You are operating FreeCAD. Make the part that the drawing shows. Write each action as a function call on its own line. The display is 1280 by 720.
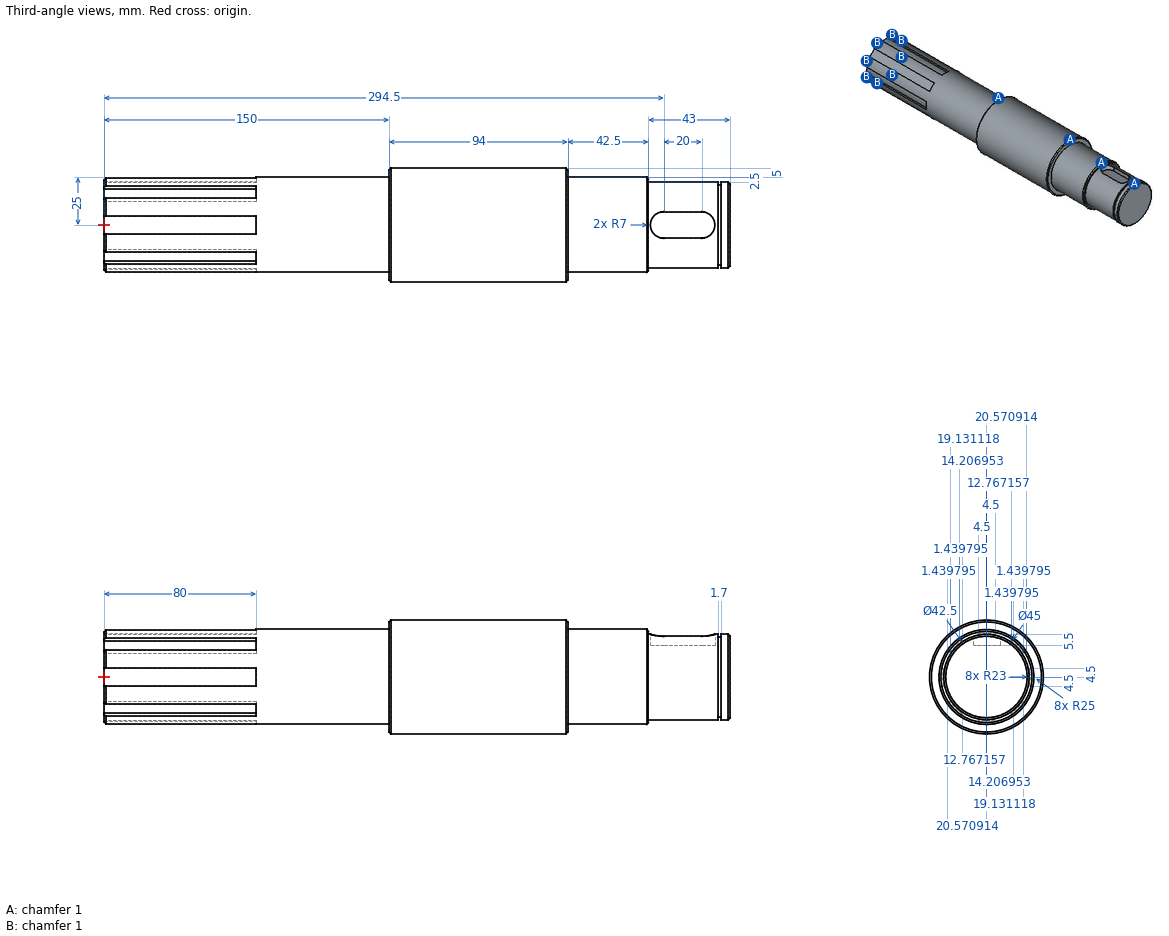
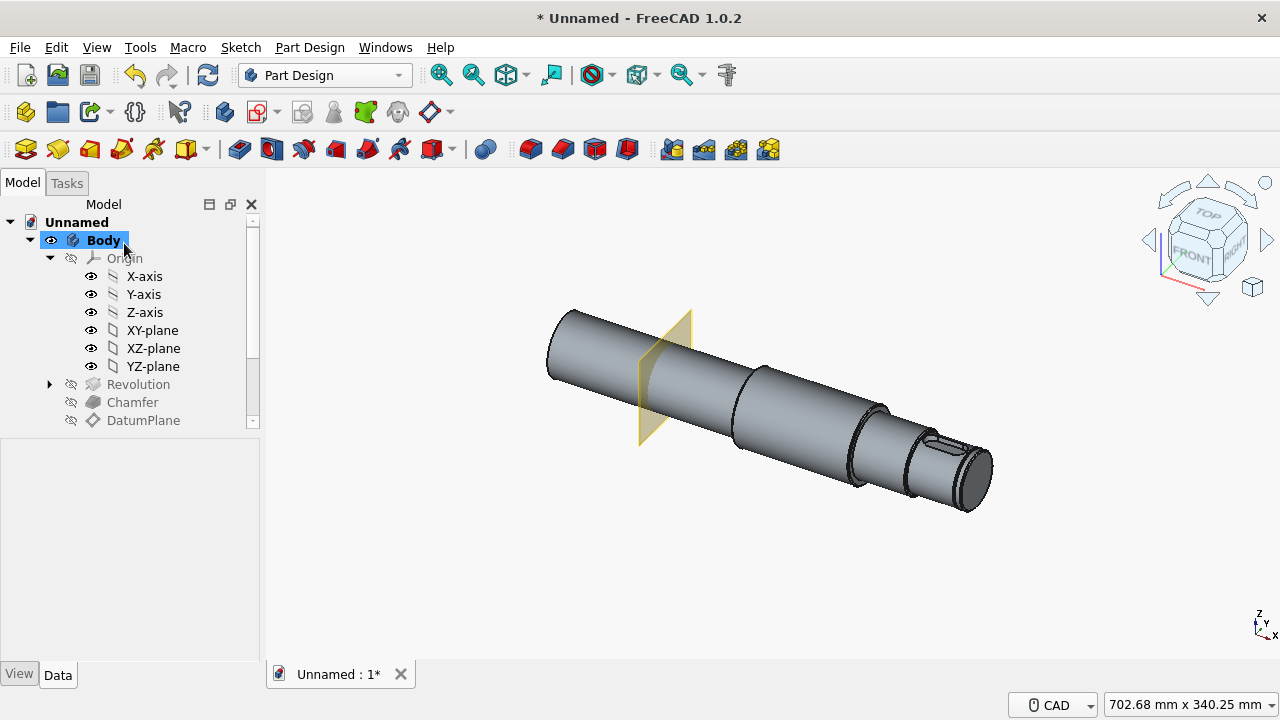
scroll(100, 326, down, 3)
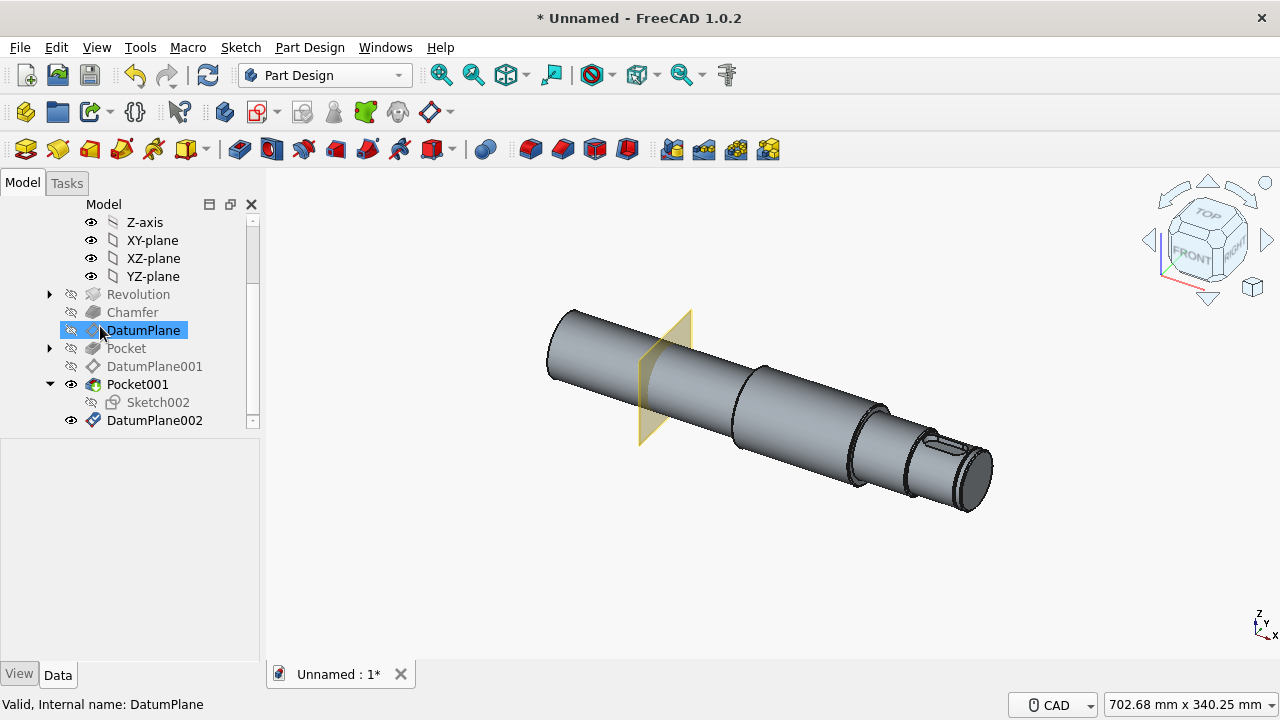
click(116, 420)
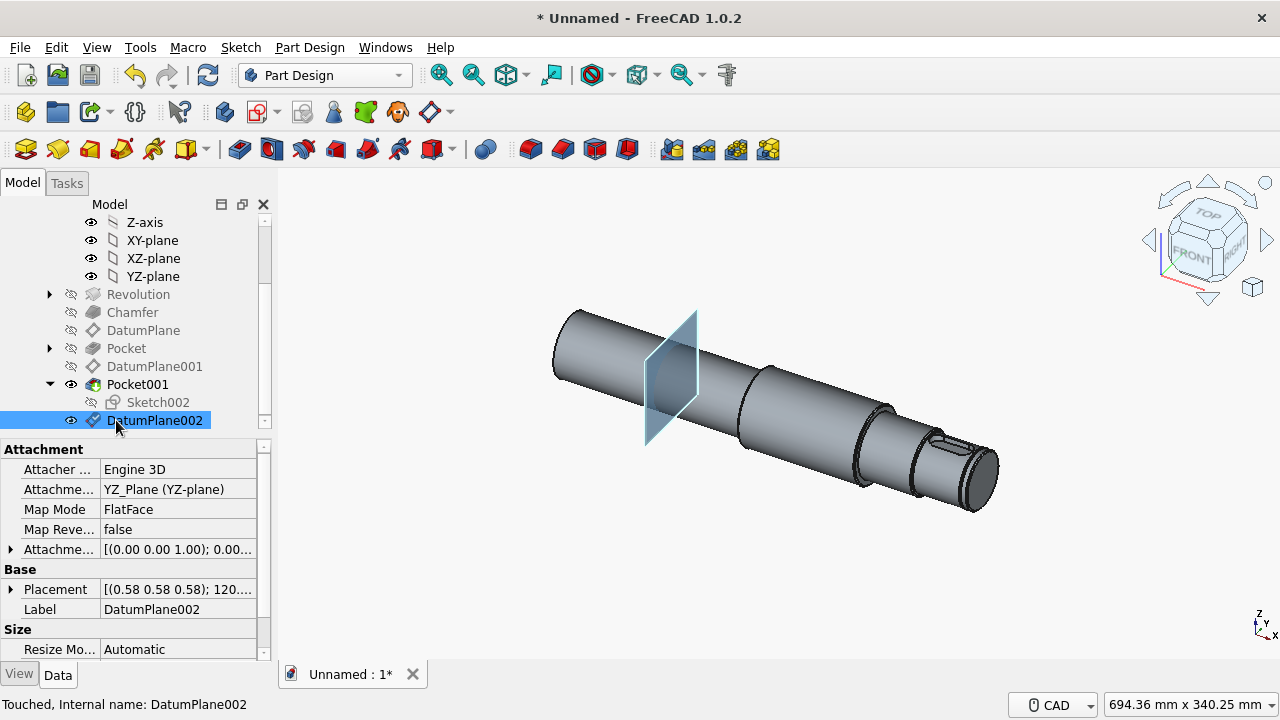
click(258, 112)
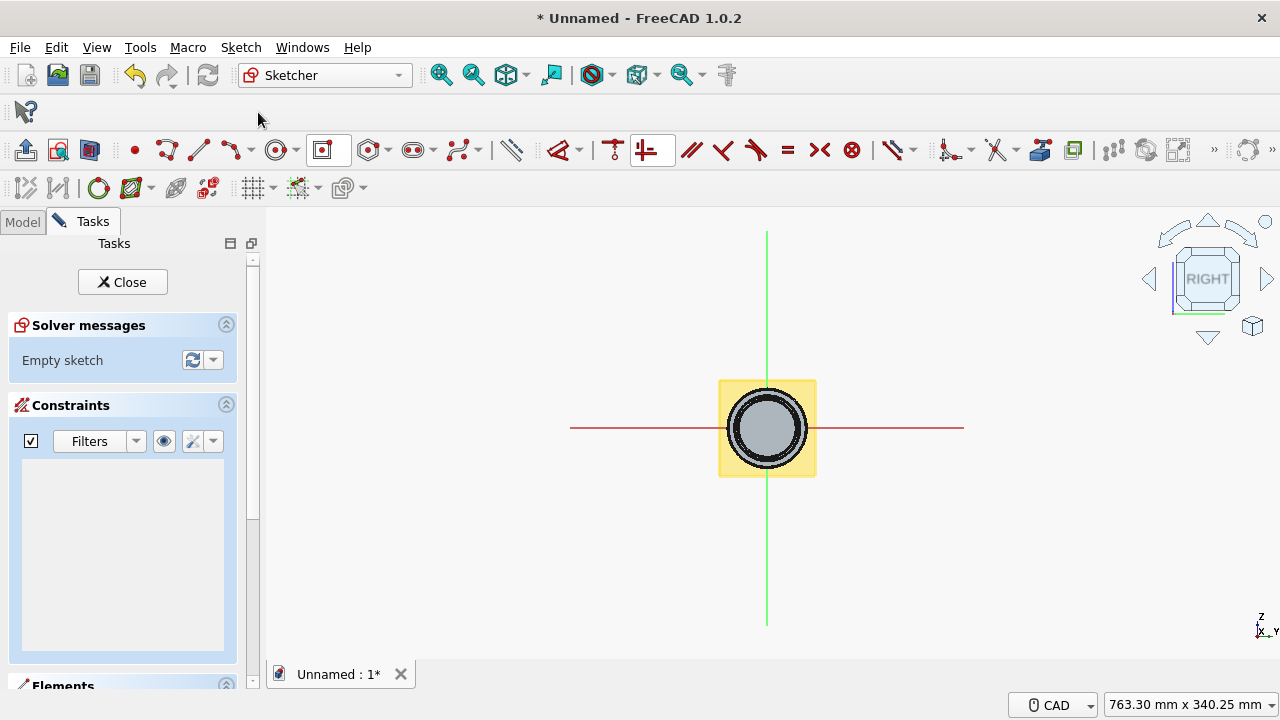
click(90, 150)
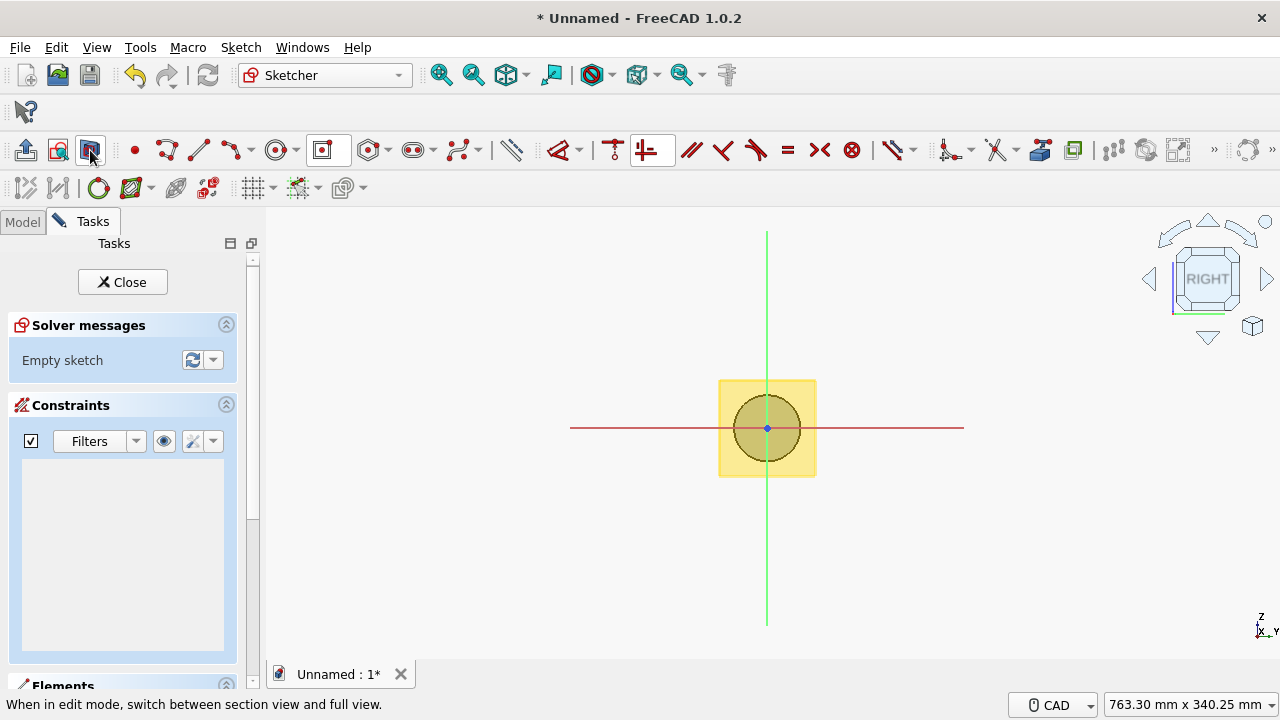
scroll(788, 427, up, 7)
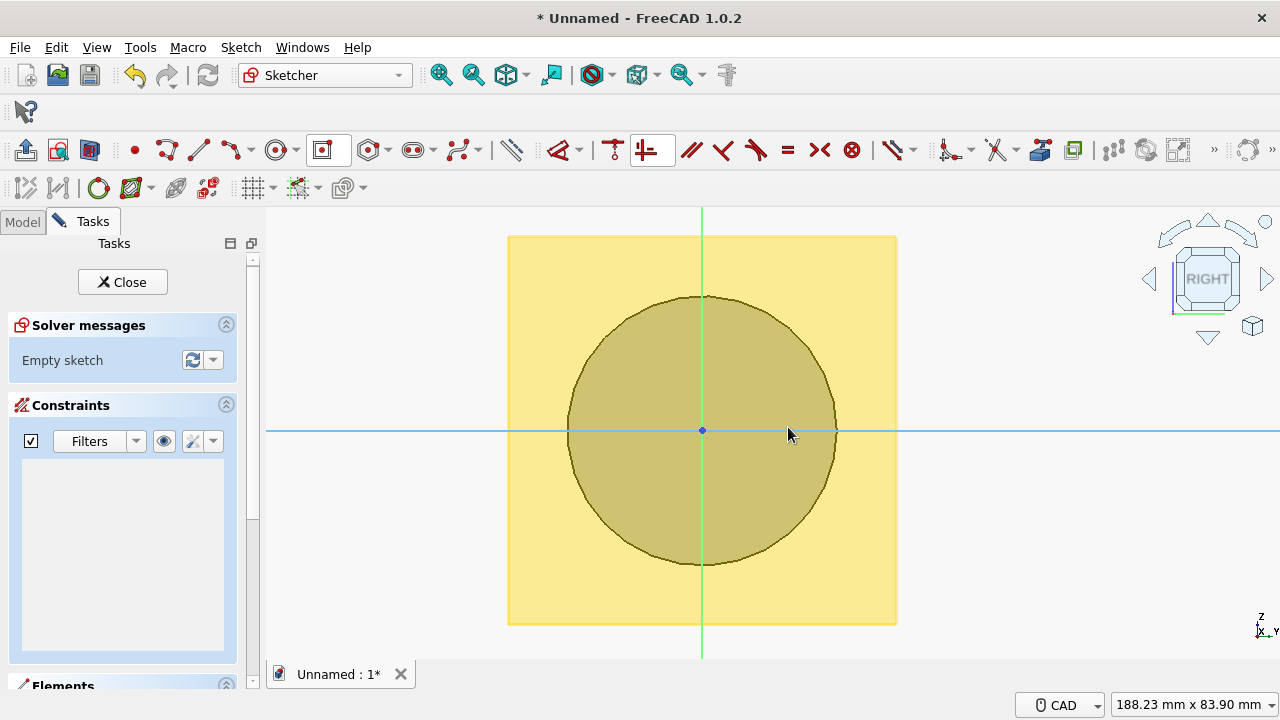
click(200, 150)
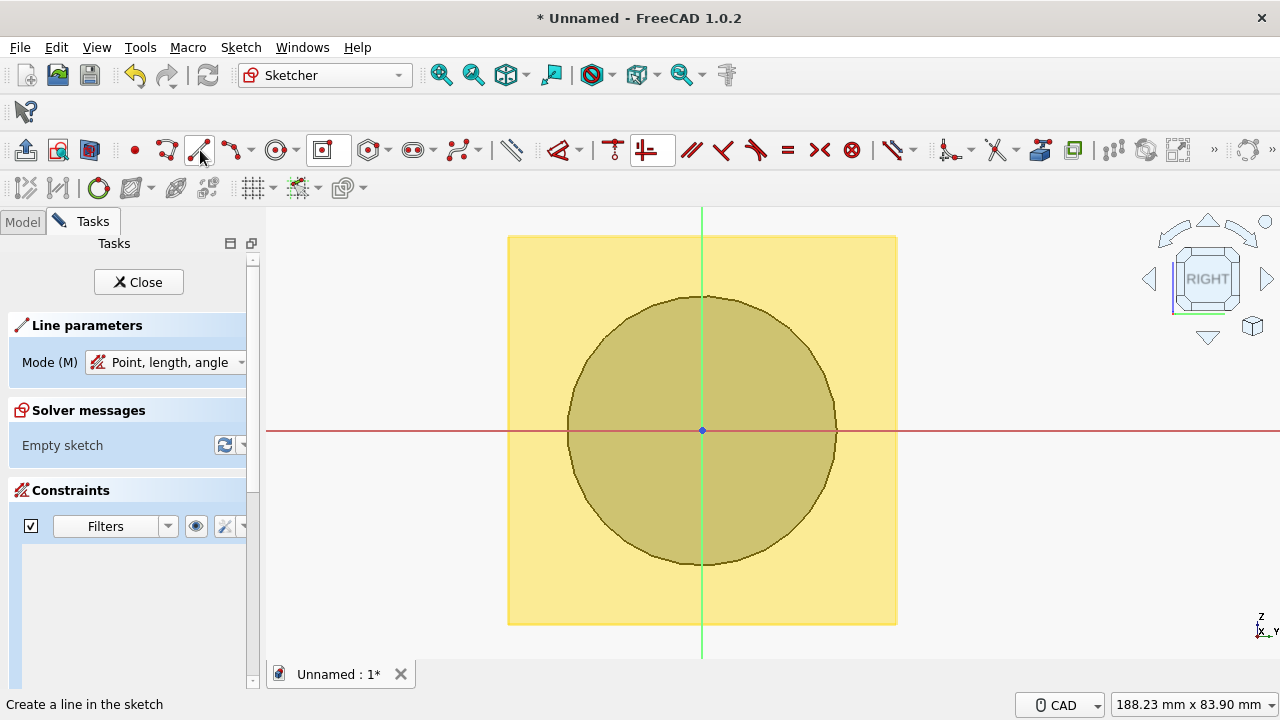
click(835, 455)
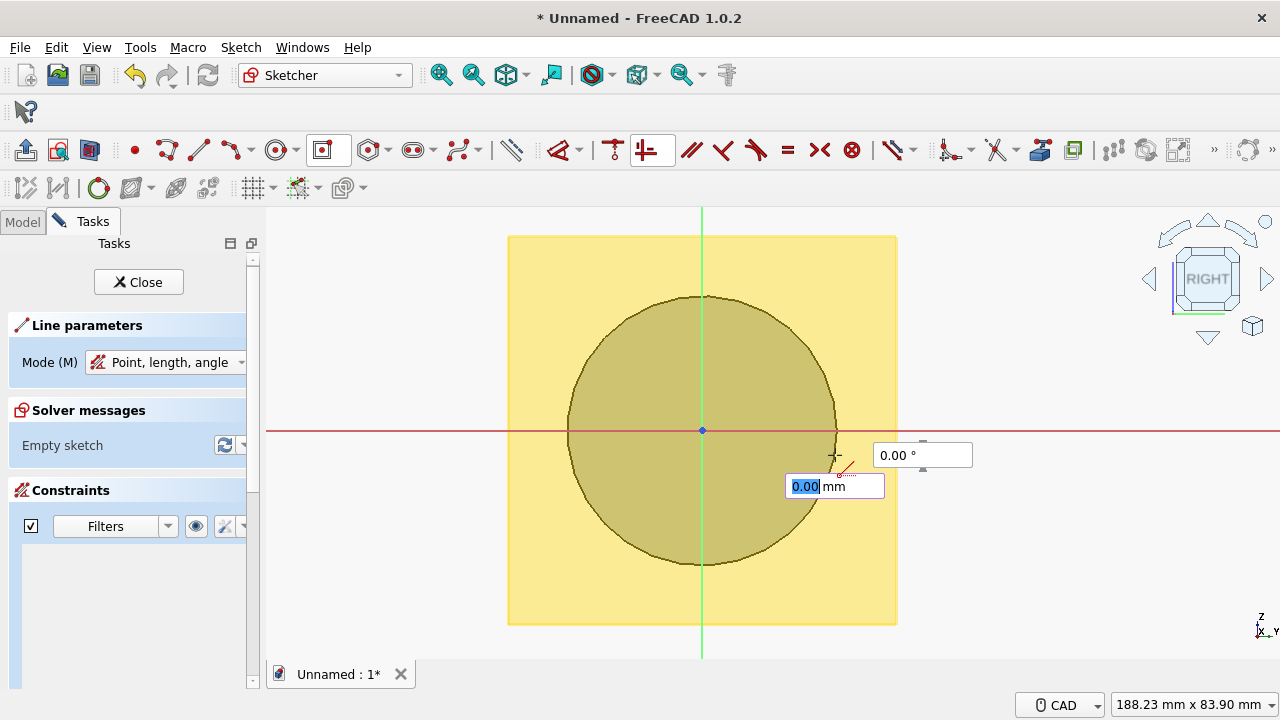
scroll(824, 455, up, 2)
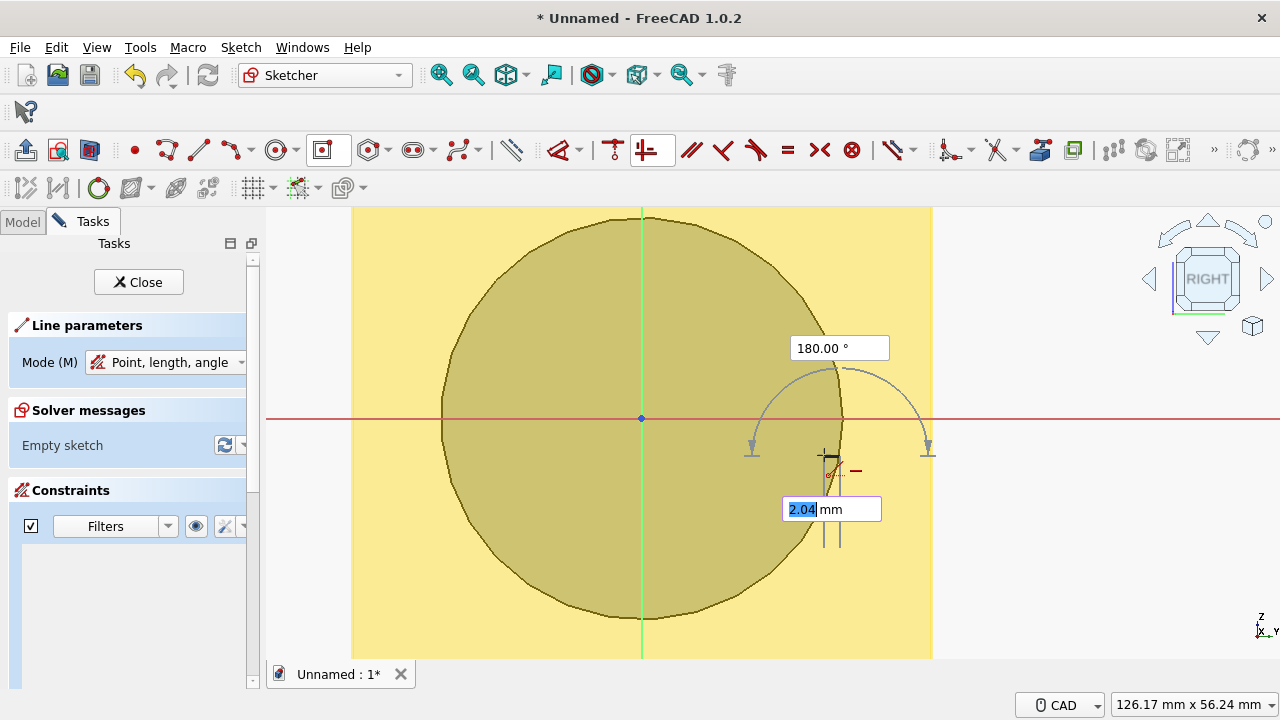
click(823, 455)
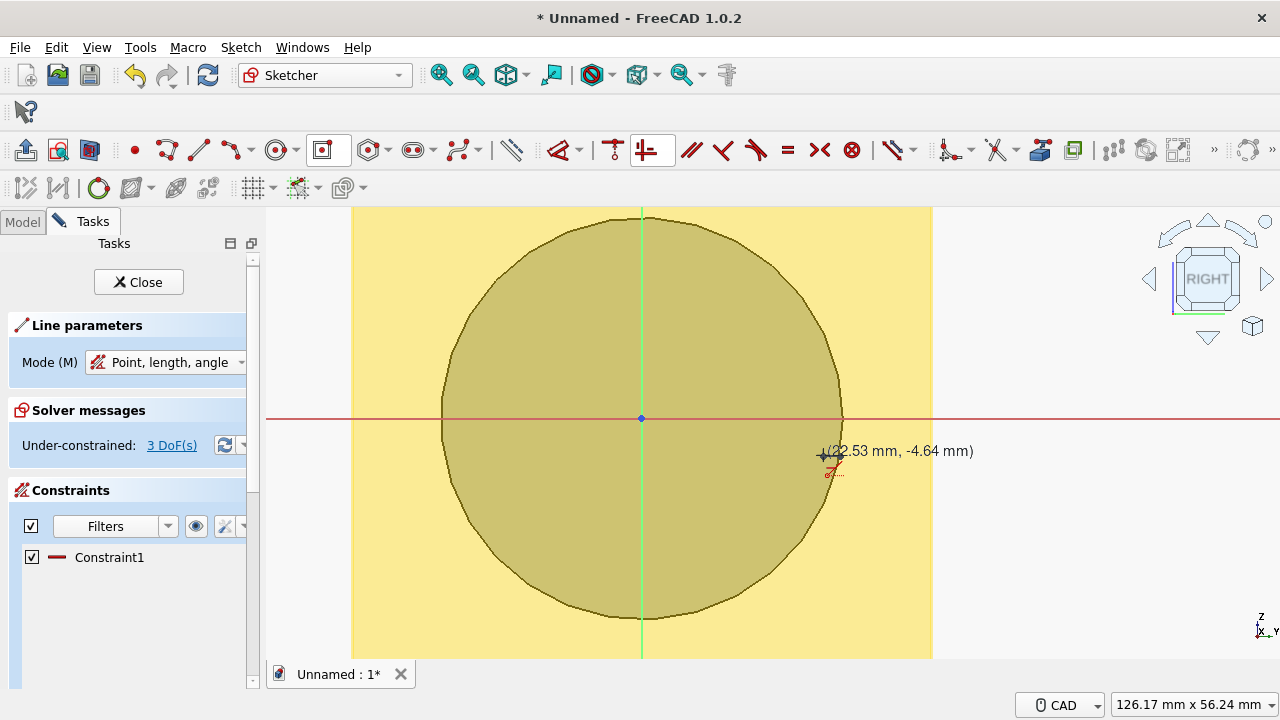
click(823, 383)
click(840, 383)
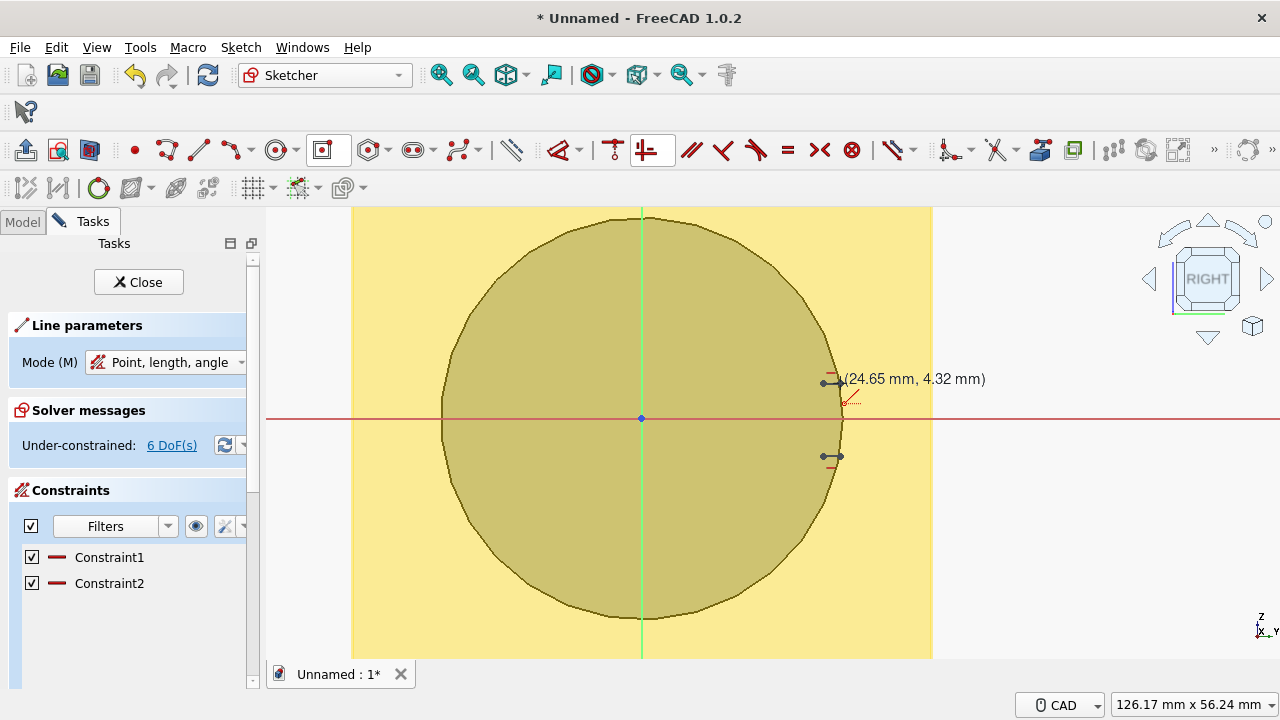
click(232, 150)